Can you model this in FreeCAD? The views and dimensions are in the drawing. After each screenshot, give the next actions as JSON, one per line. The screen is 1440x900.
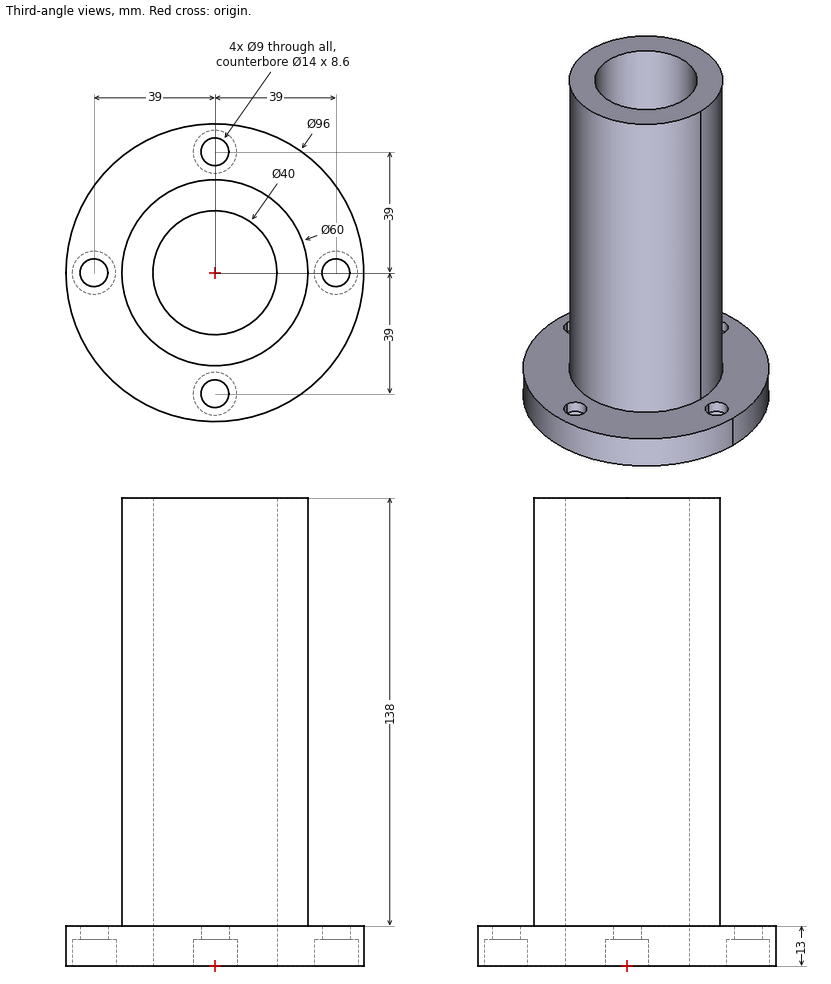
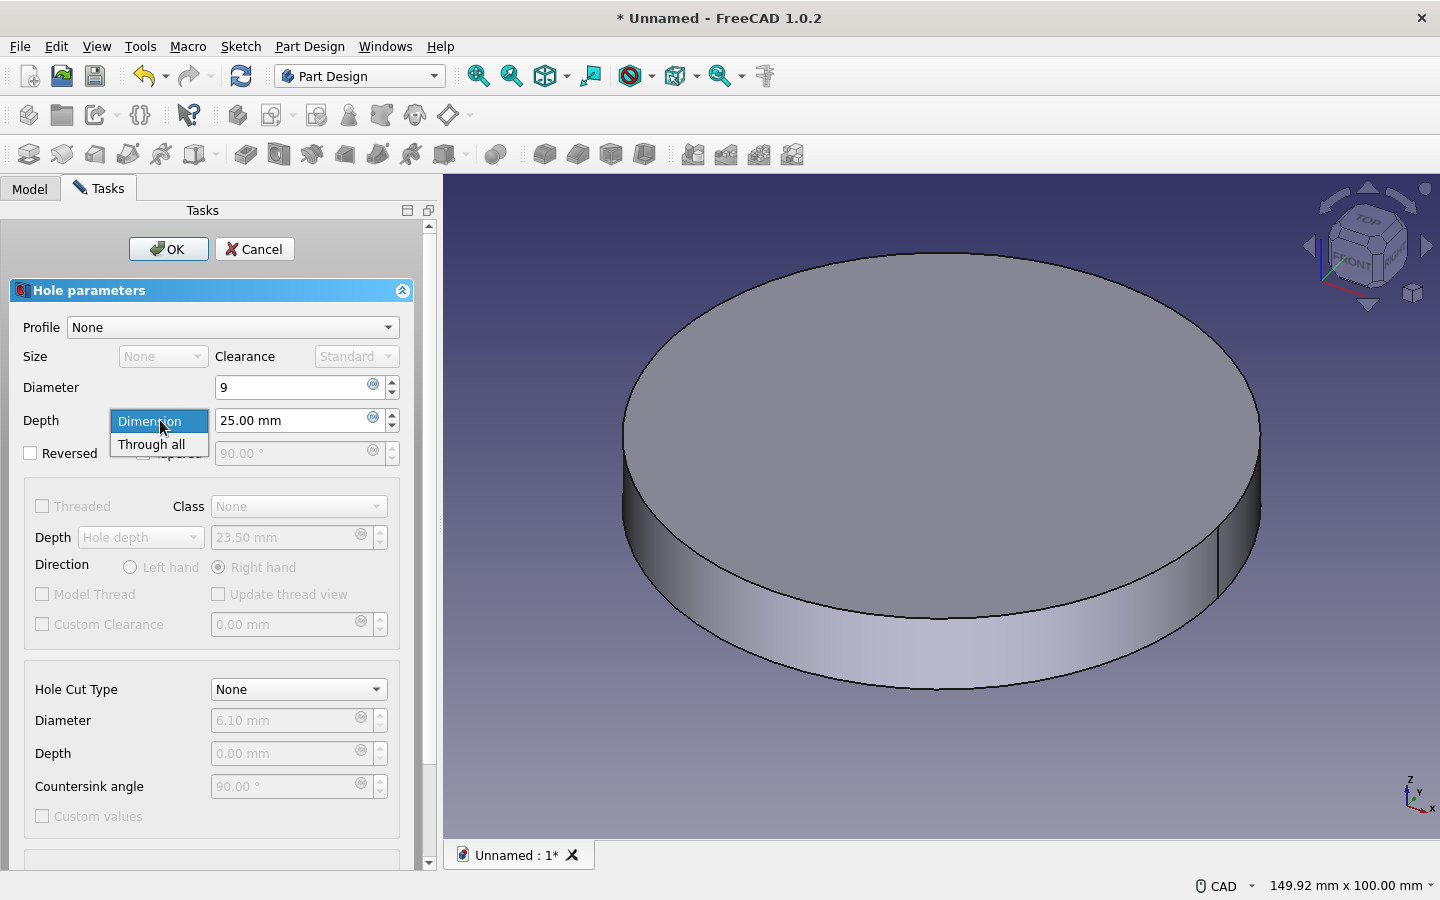
{"action": "left_click", "coordinate": [158, 444]}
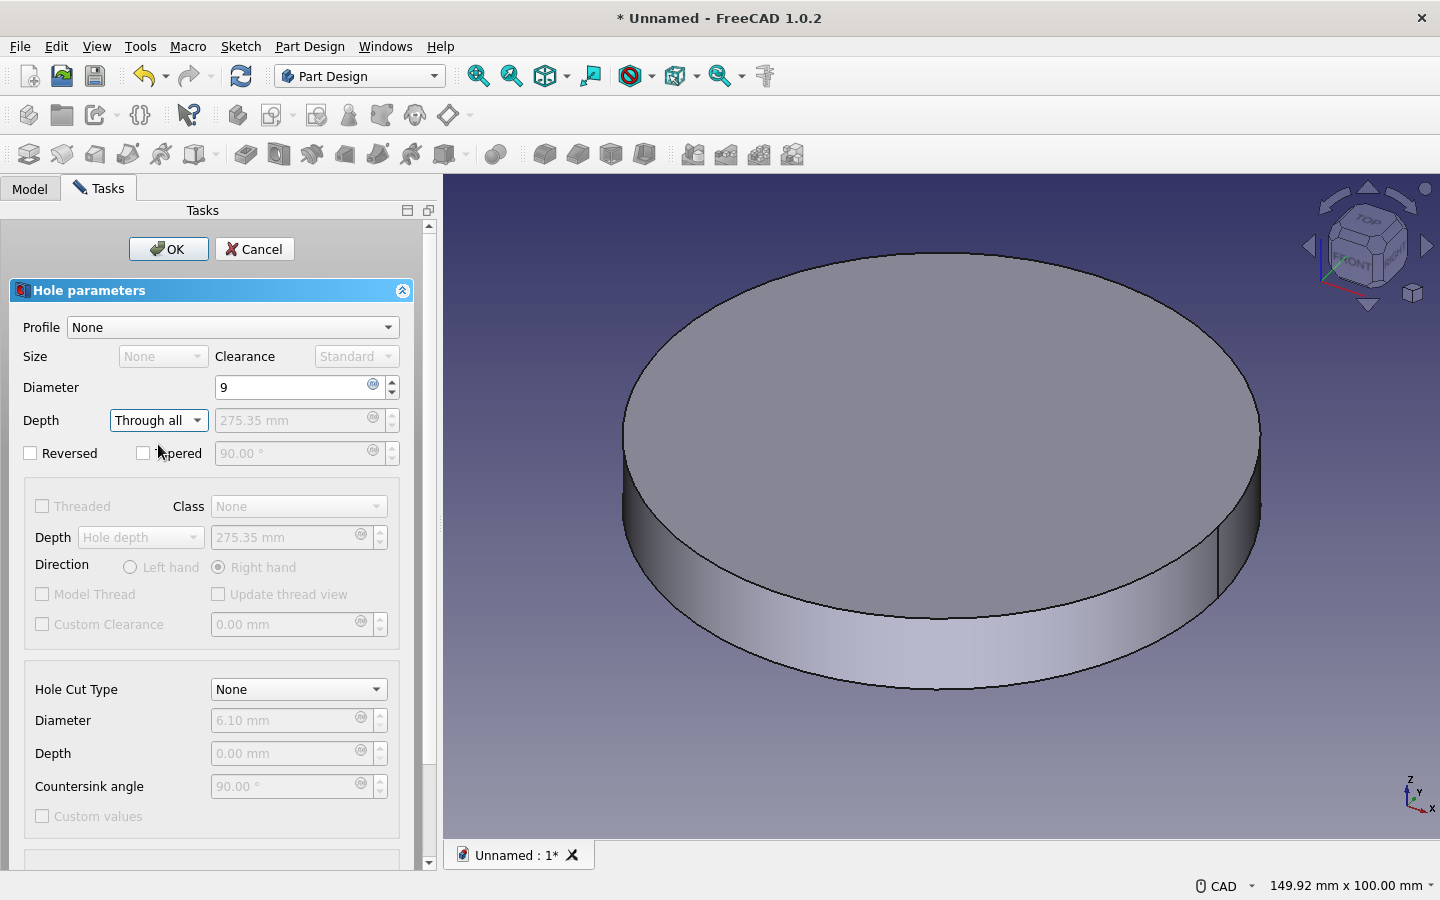
{"action": "left_click", "coordinate": [31, 453]}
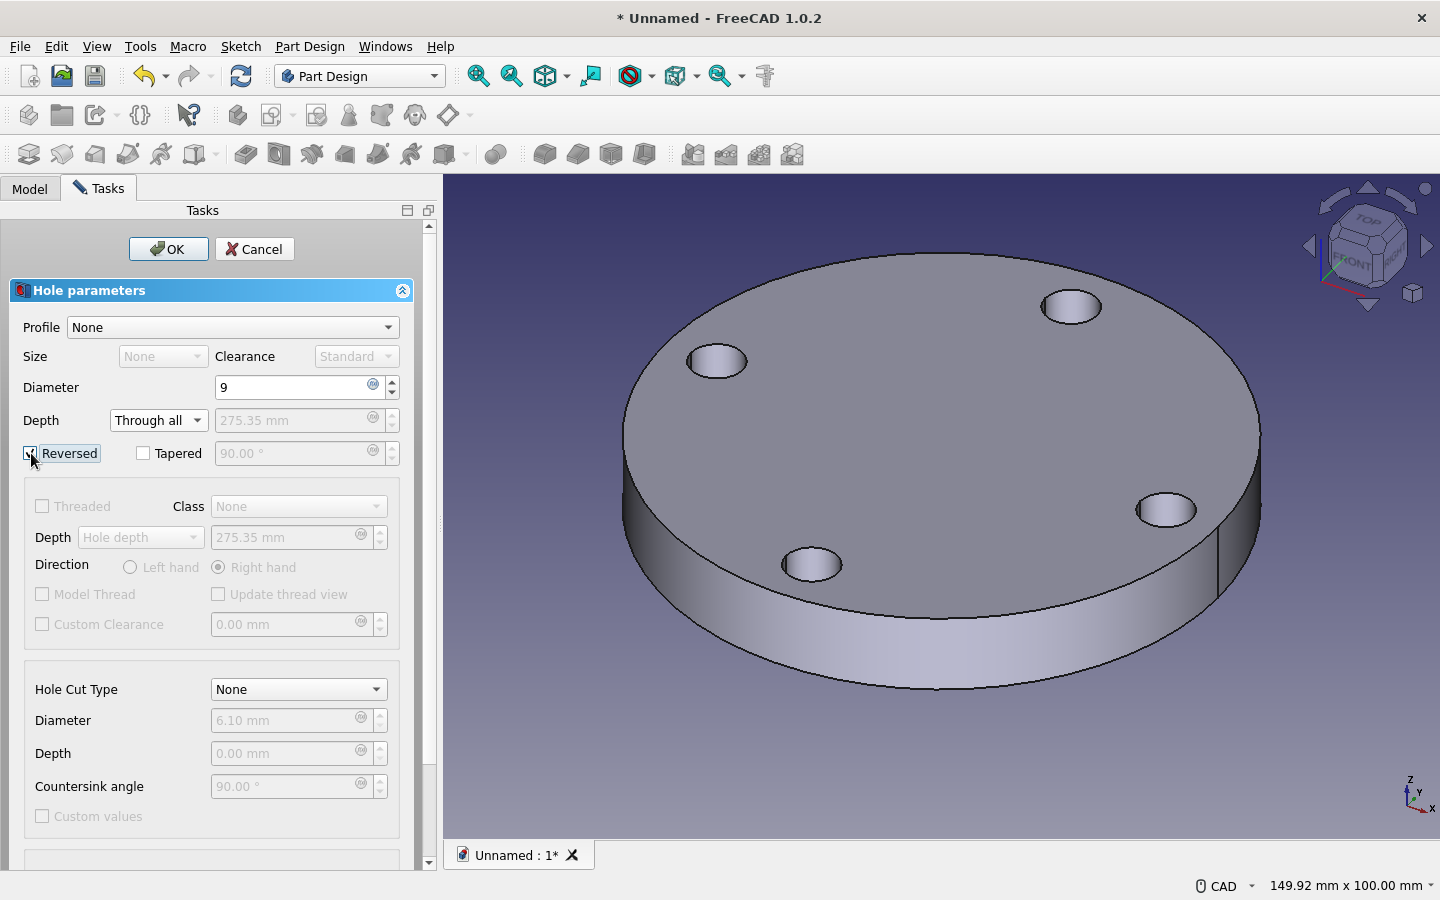
{"action": "left_click", "coordinate": [300, 690]}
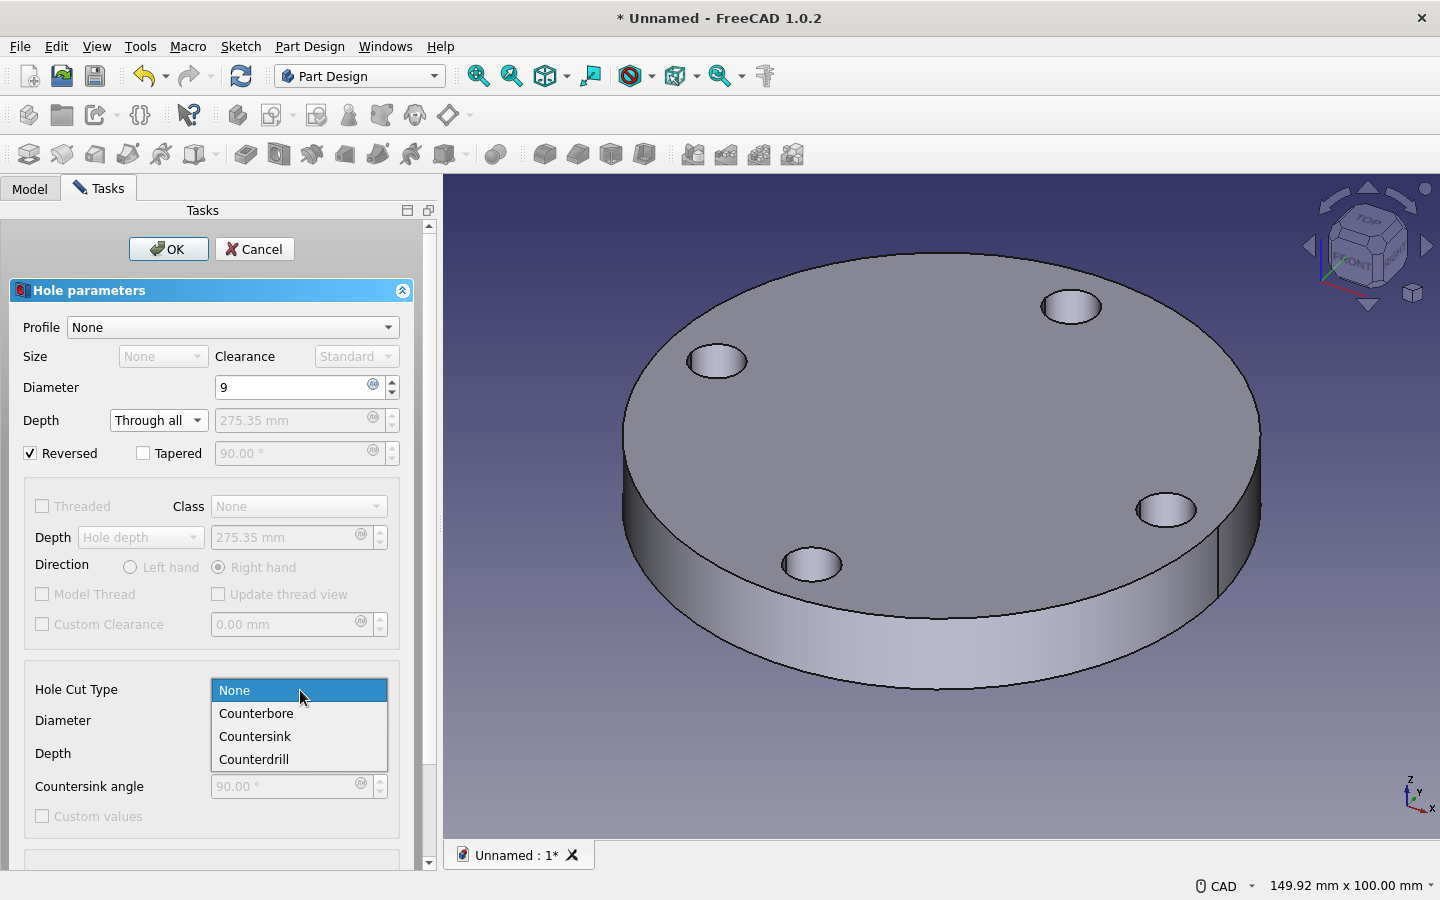
{"action": "left_click", "coordinate": [298, 714]}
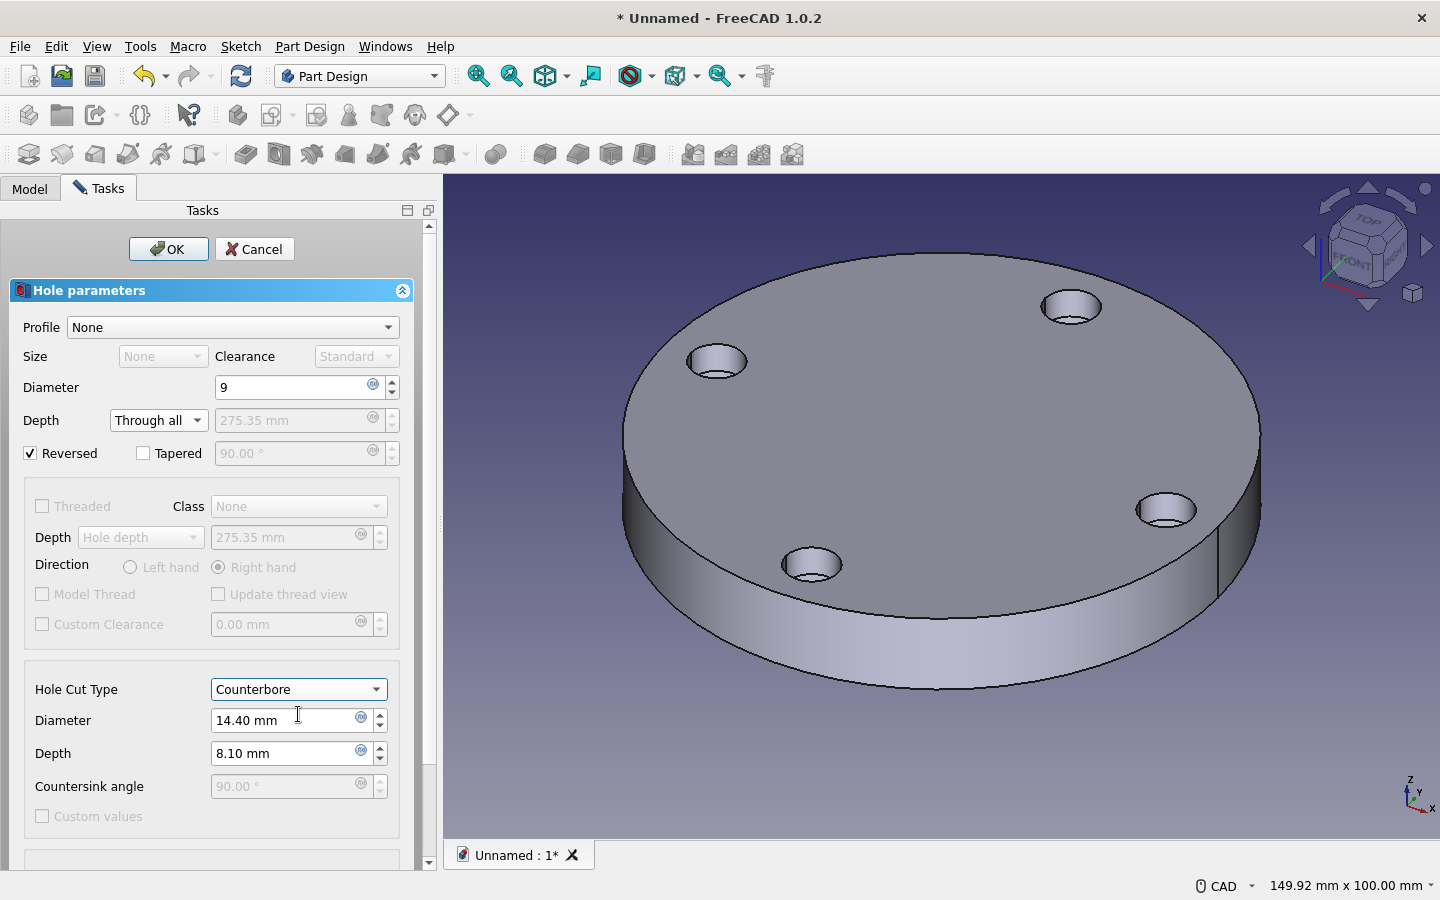
{"action": "triple_click", "coordinate": [292, 720]}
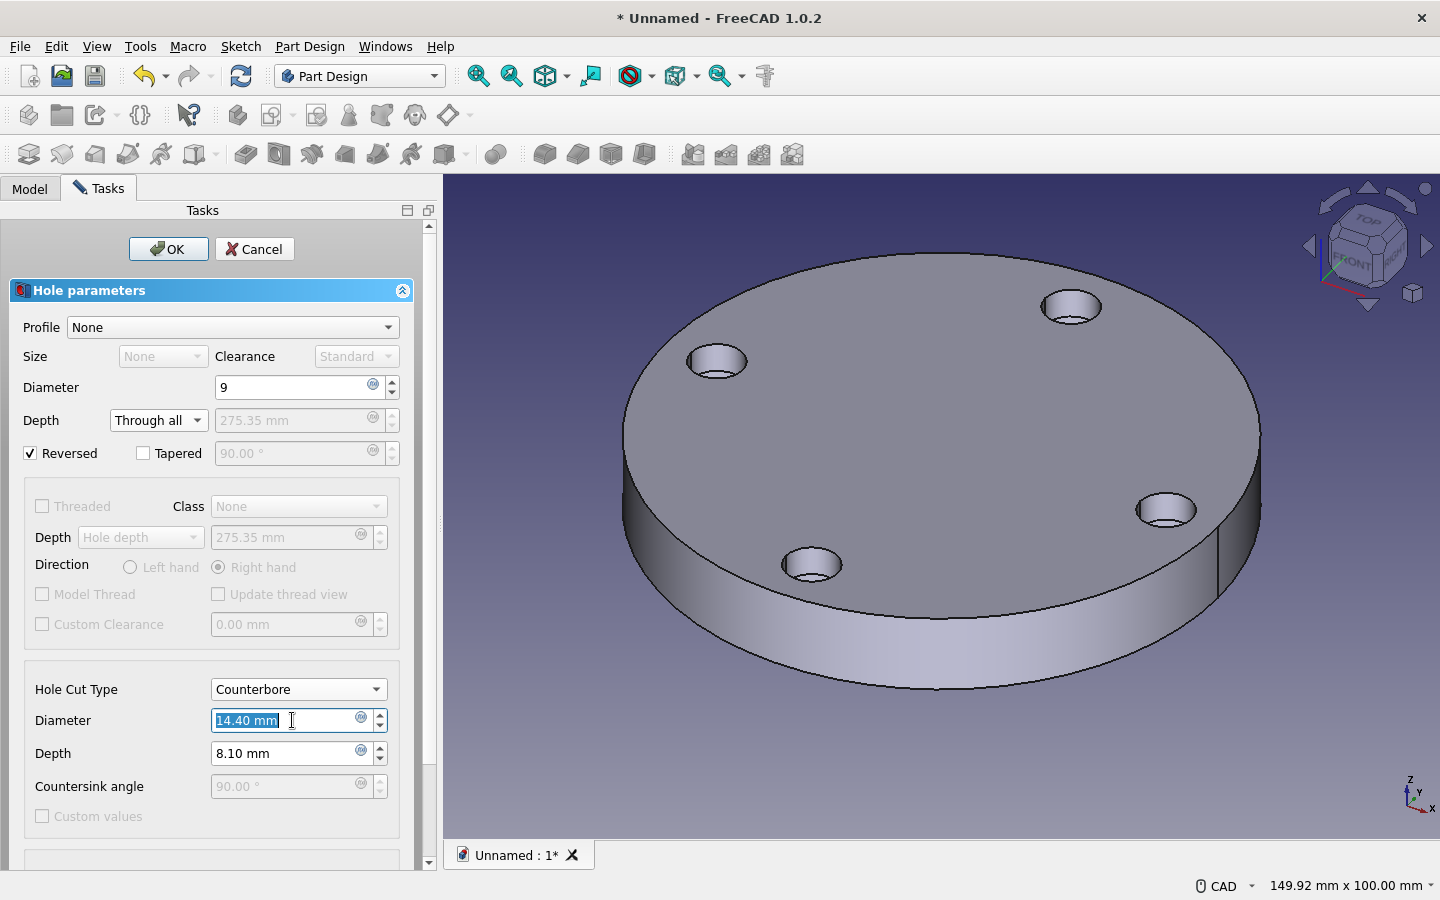
{"action": "type", "text": "14"}
{"action": "key", "text": "Tab"}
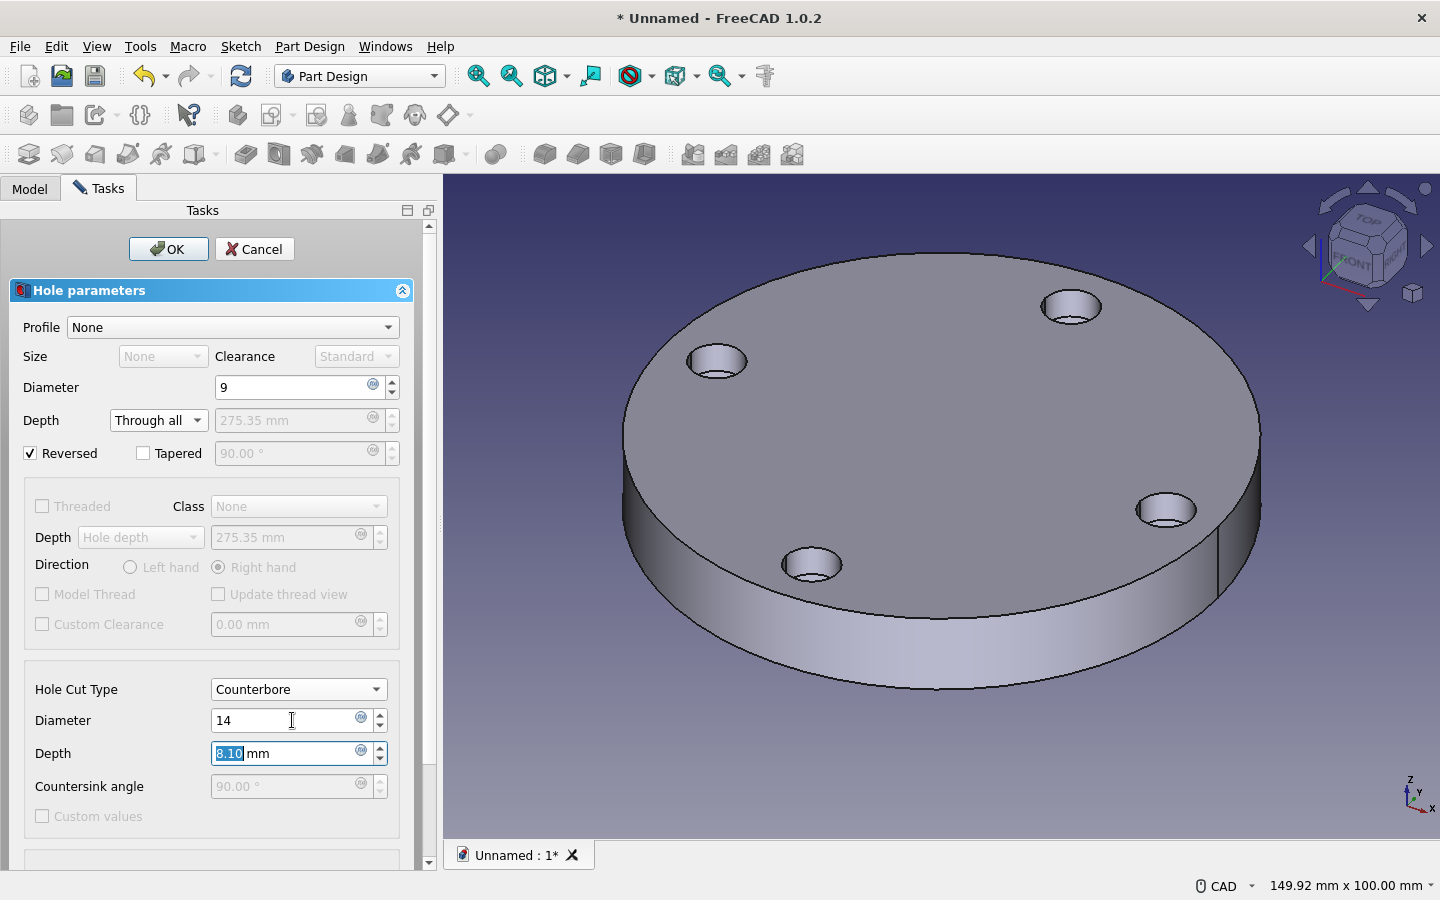
{"action": "type", "text": "8.6"}
{"action": "key", "text": "Tab"}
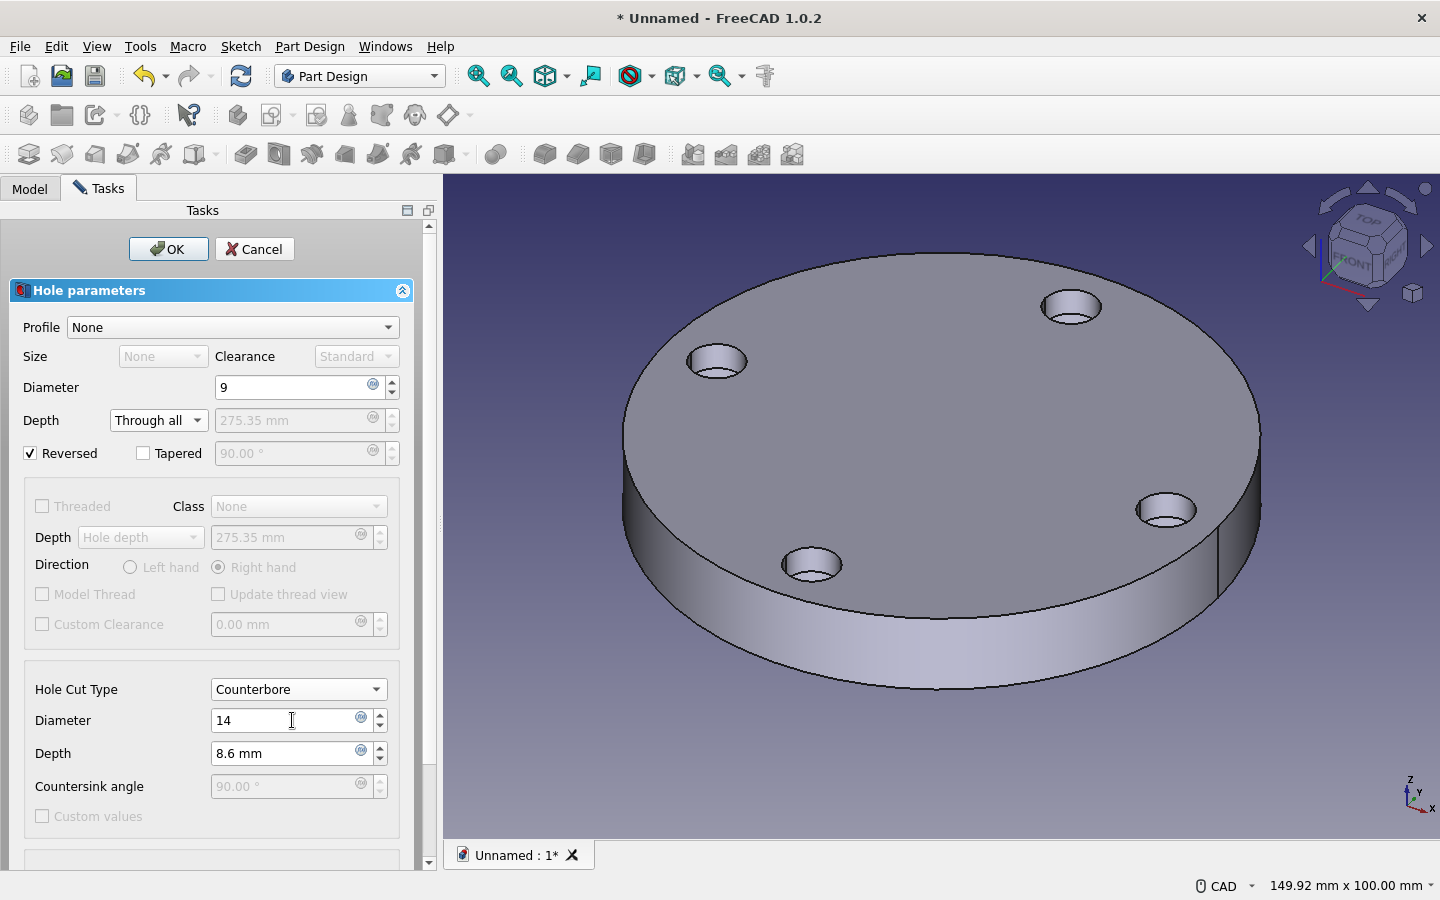
{"action": "left_click", "coordinate": [169, 249]}